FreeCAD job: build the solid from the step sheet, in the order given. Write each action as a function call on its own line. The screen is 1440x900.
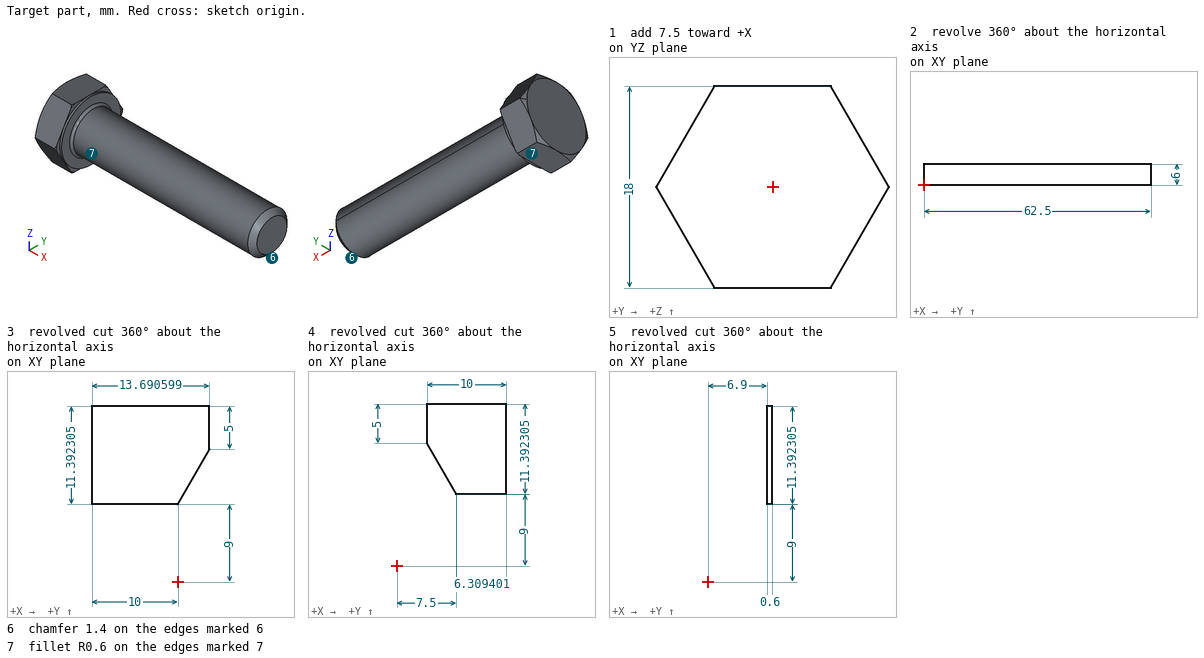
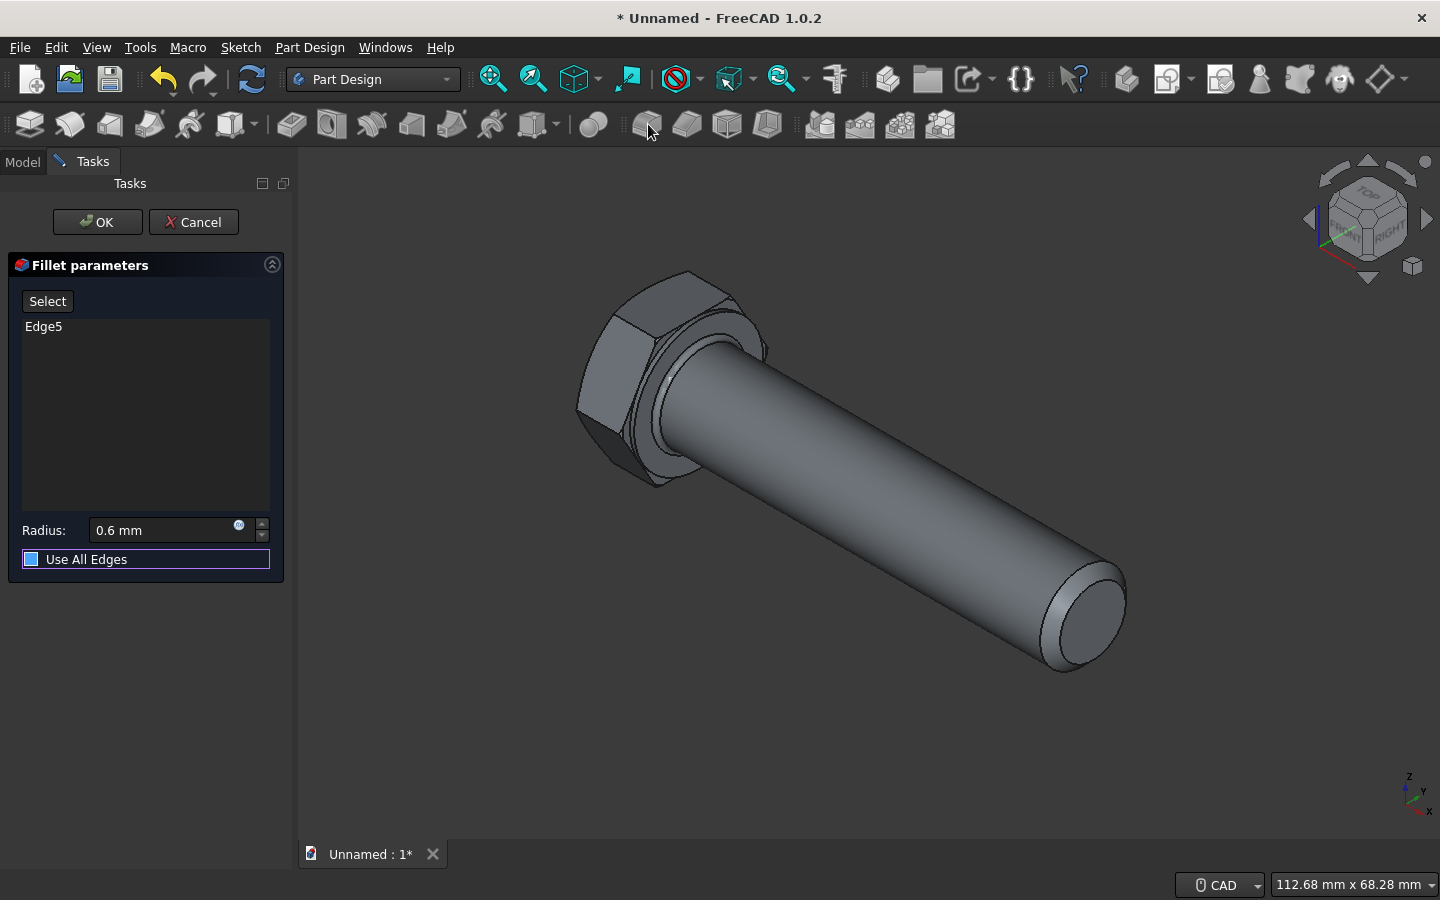
click(98, 222)